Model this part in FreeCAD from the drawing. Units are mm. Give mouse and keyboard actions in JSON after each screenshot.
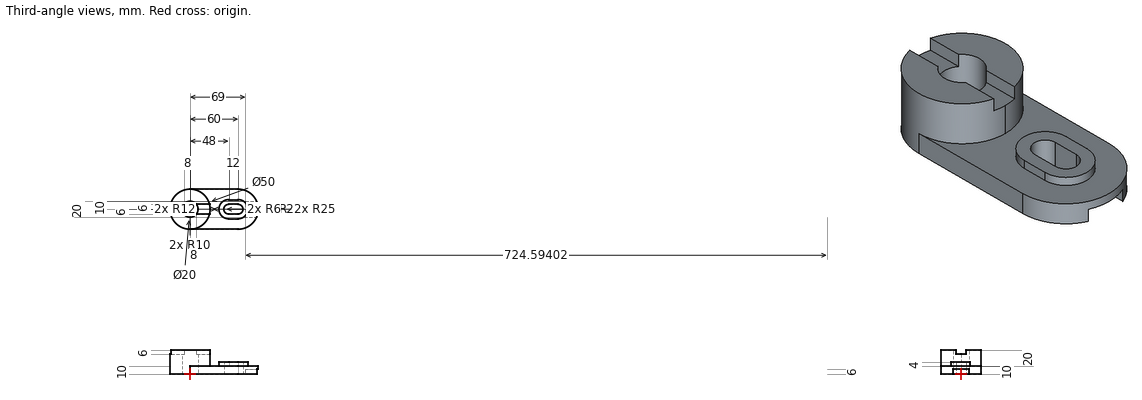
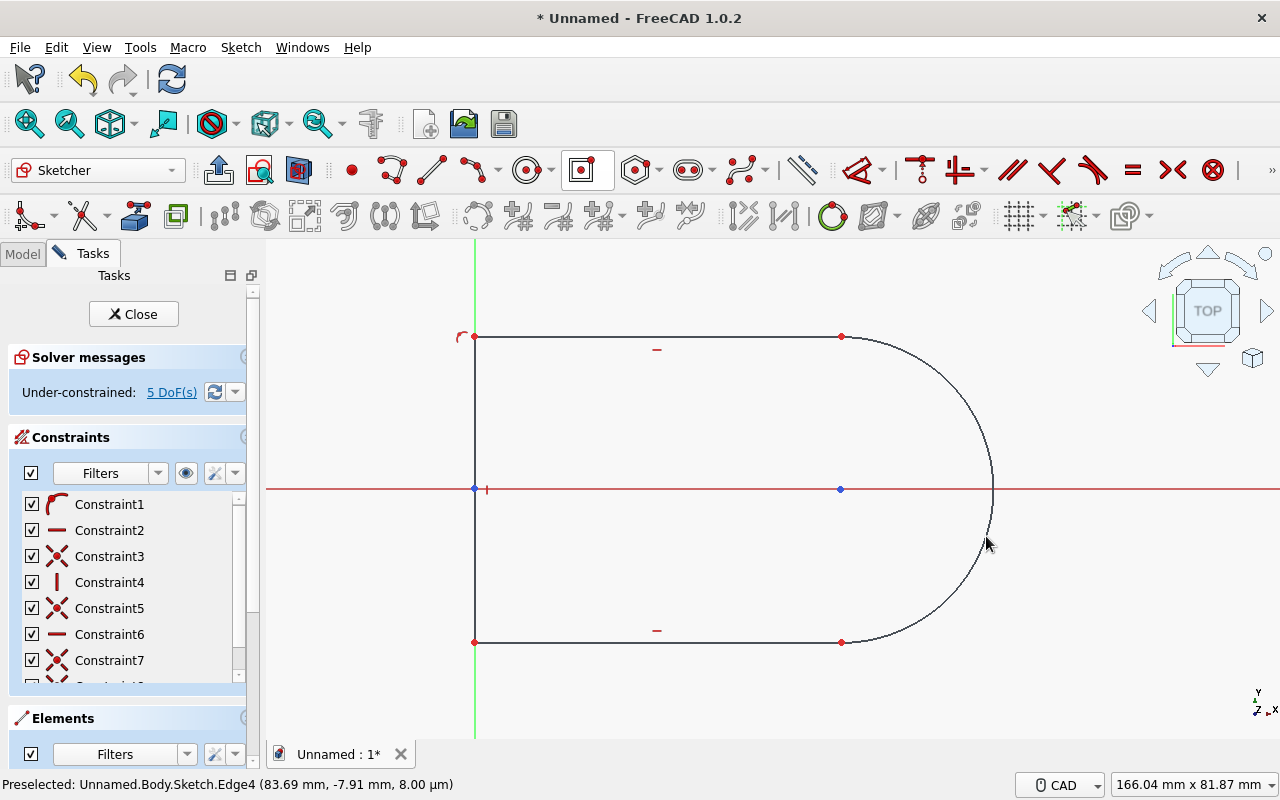
{"action": "left_click", "coordinate": [731, 337]}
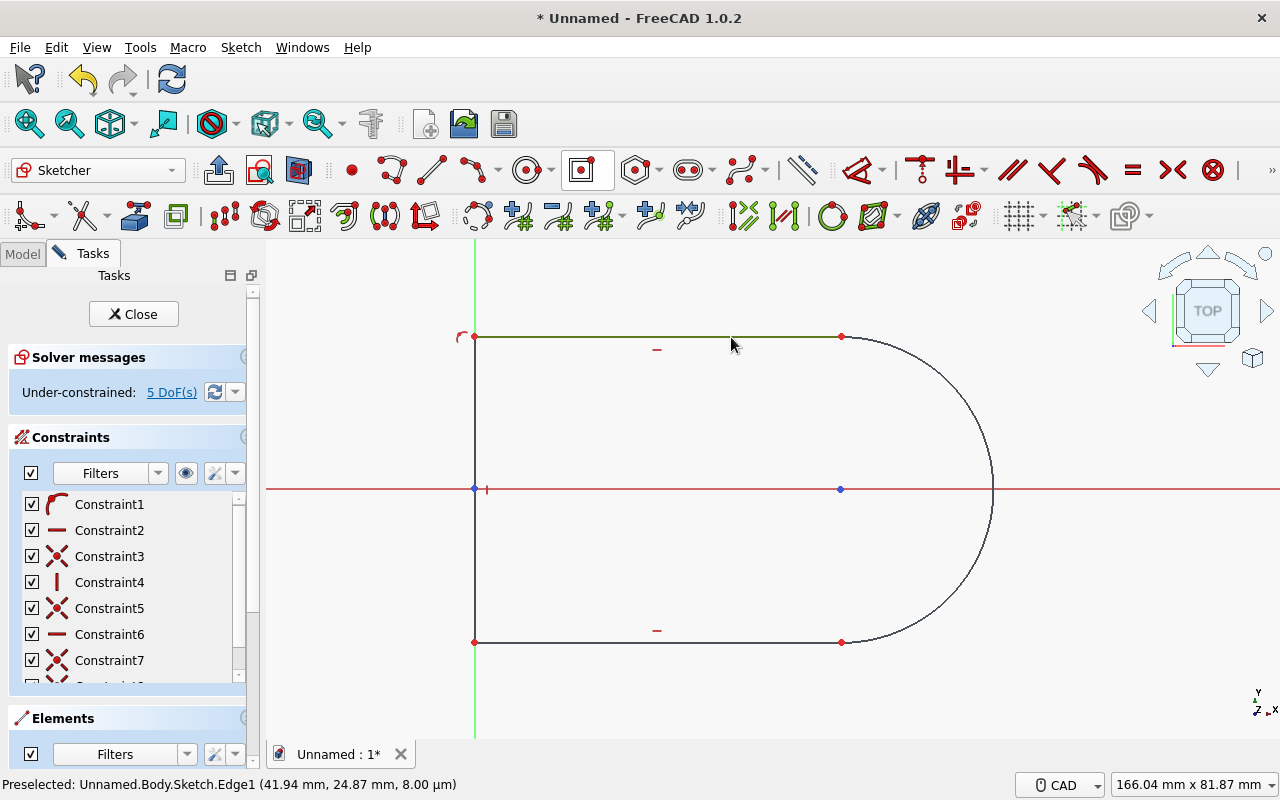
{"action": "left_click", "coordinate": [964, 580]}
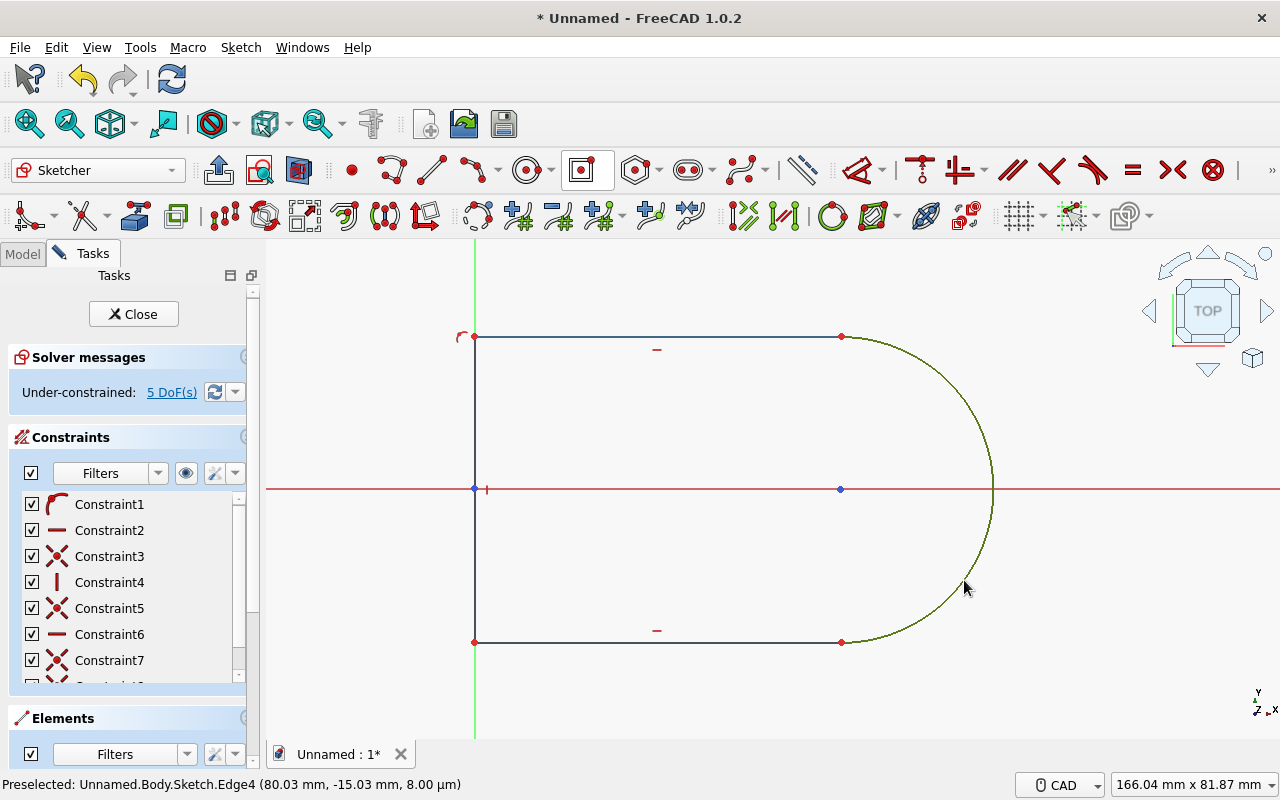
{"action": "left_click", "coordinate": [1094, 170]}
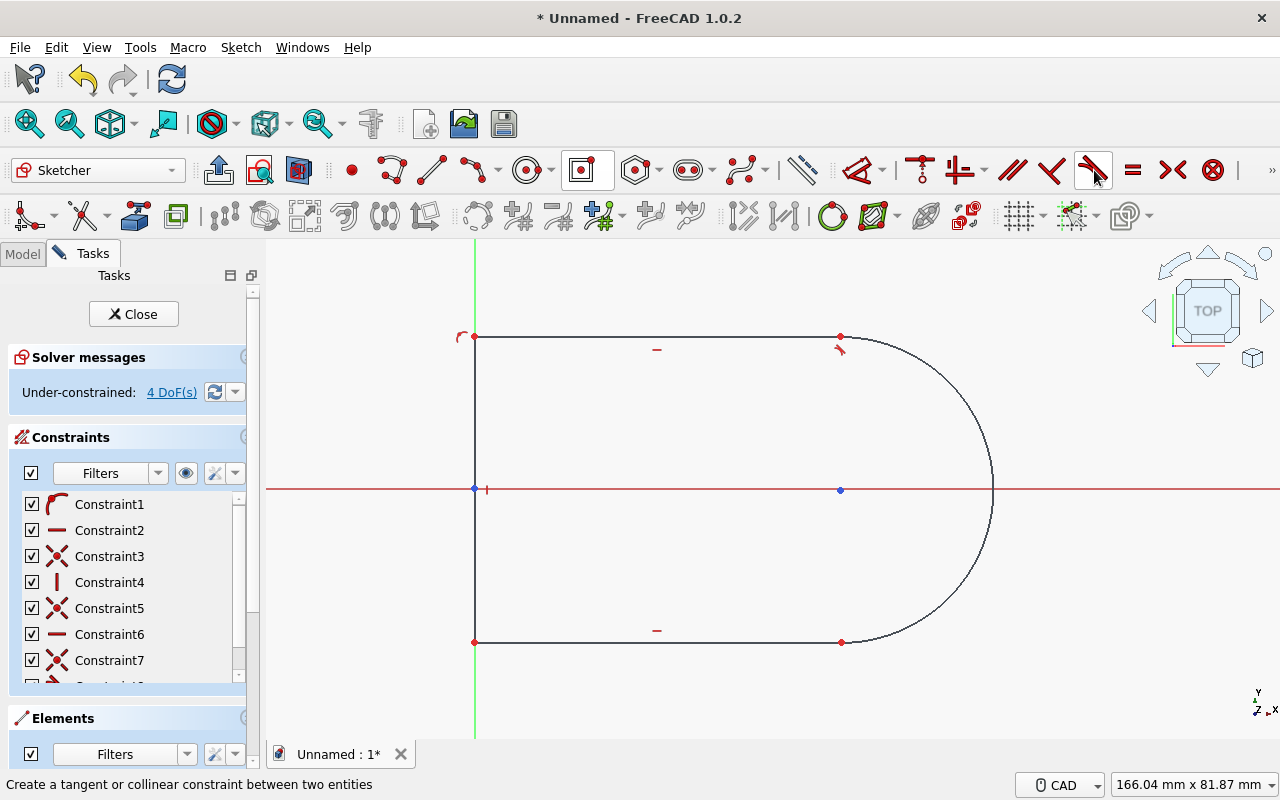
{"action": "left_click", "coordinate": [585, 643]}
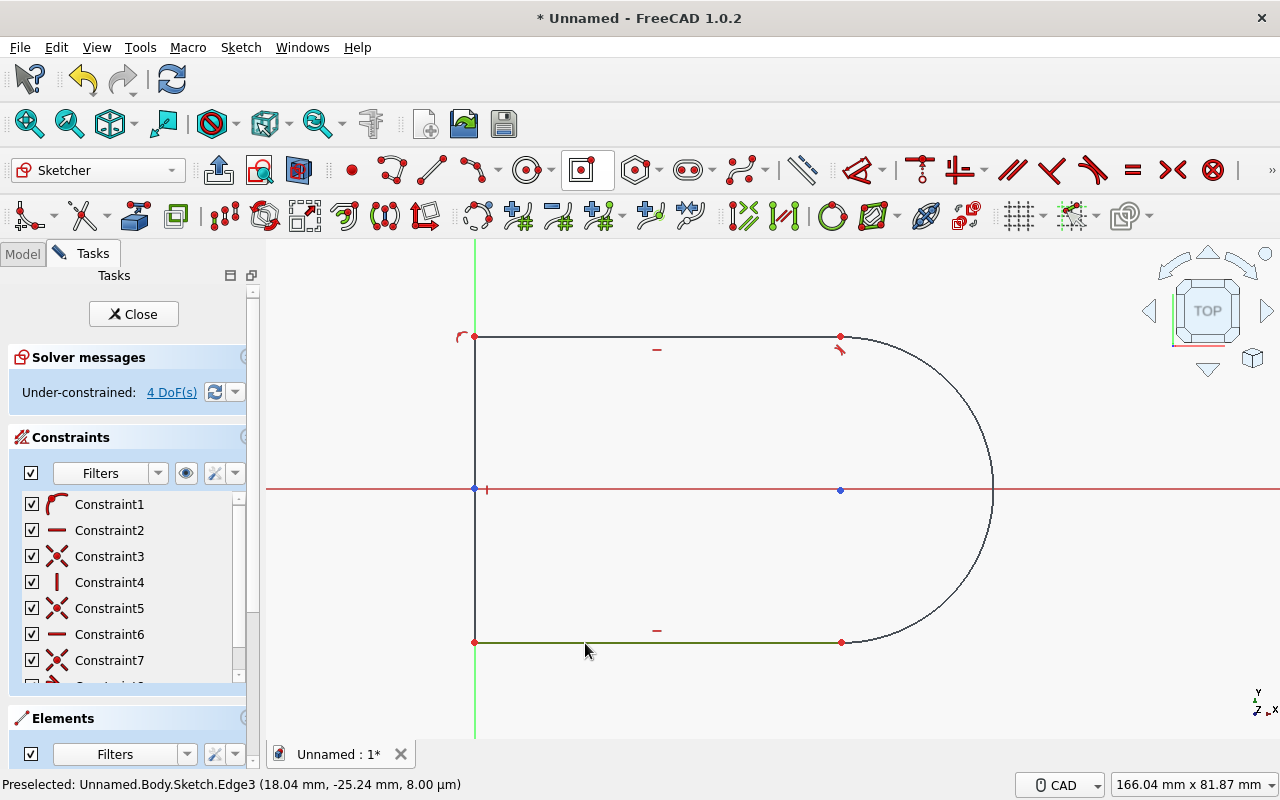
{"action": "left_click", "coordinate": [964, 580]}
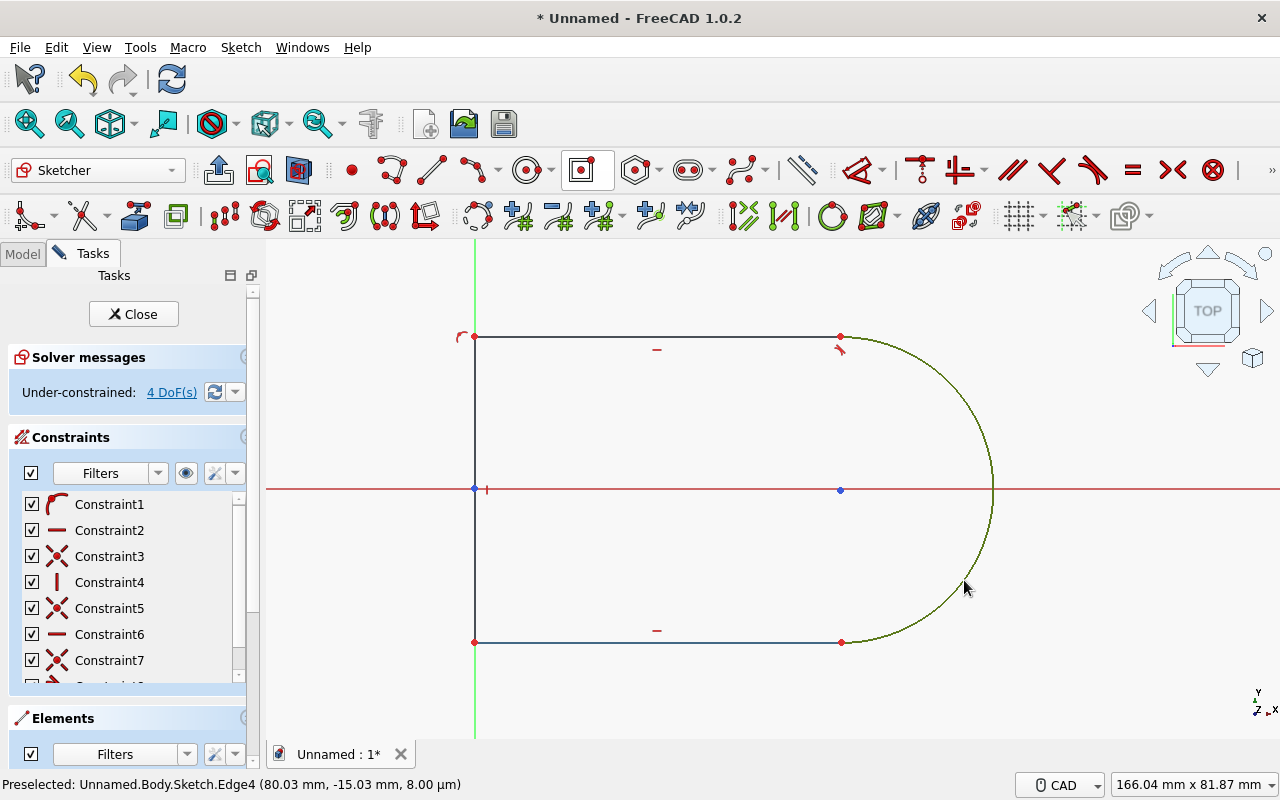
{"action": "left_click", "coordinate": [1094, 170]}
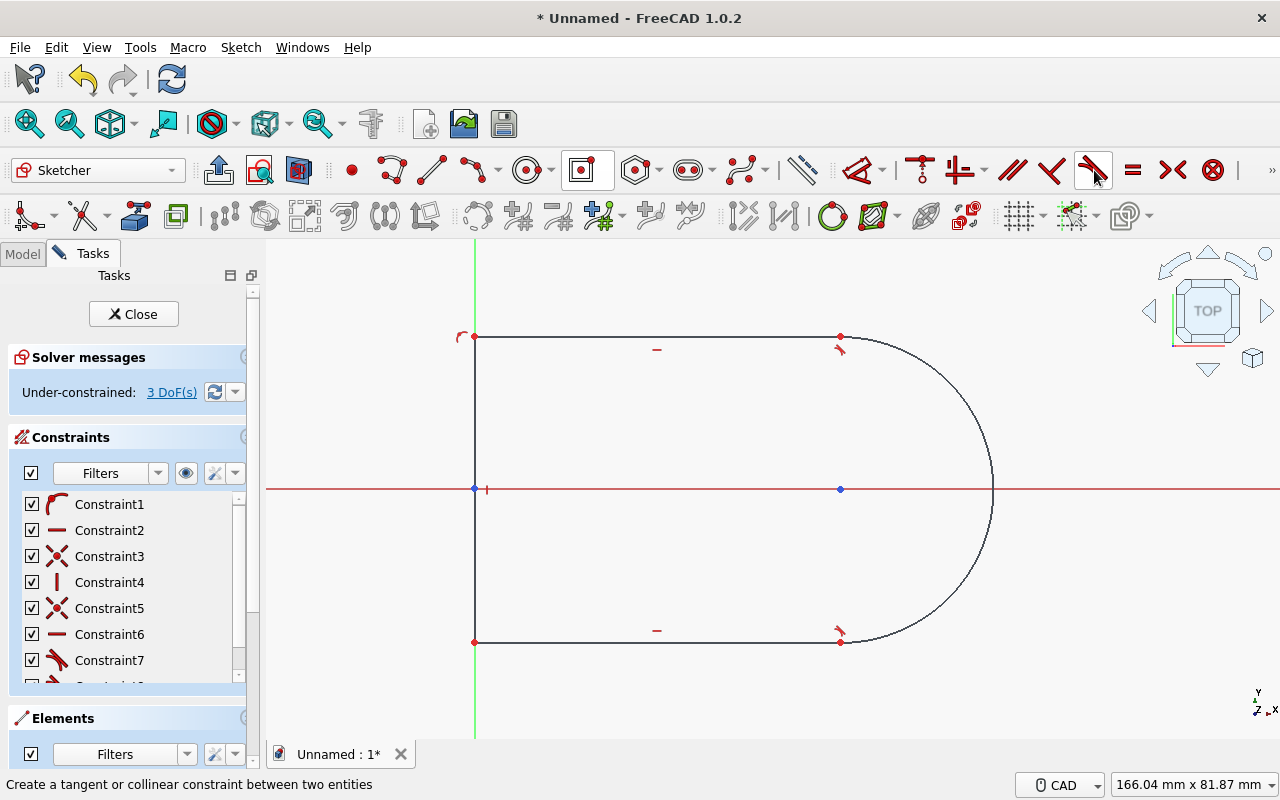
{"action": "left_click", "coordinate": [840, 490]}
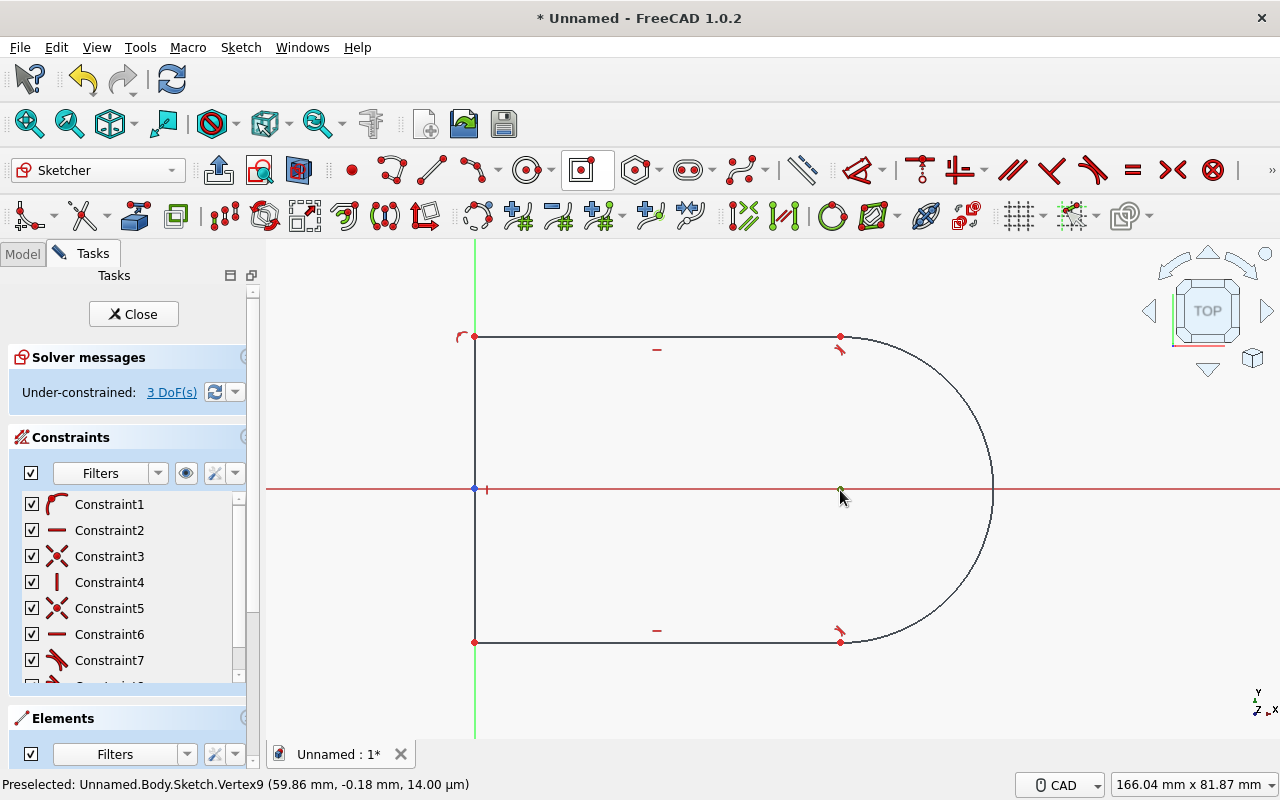
{"action": "left_click", "coordinate": [353, 489]}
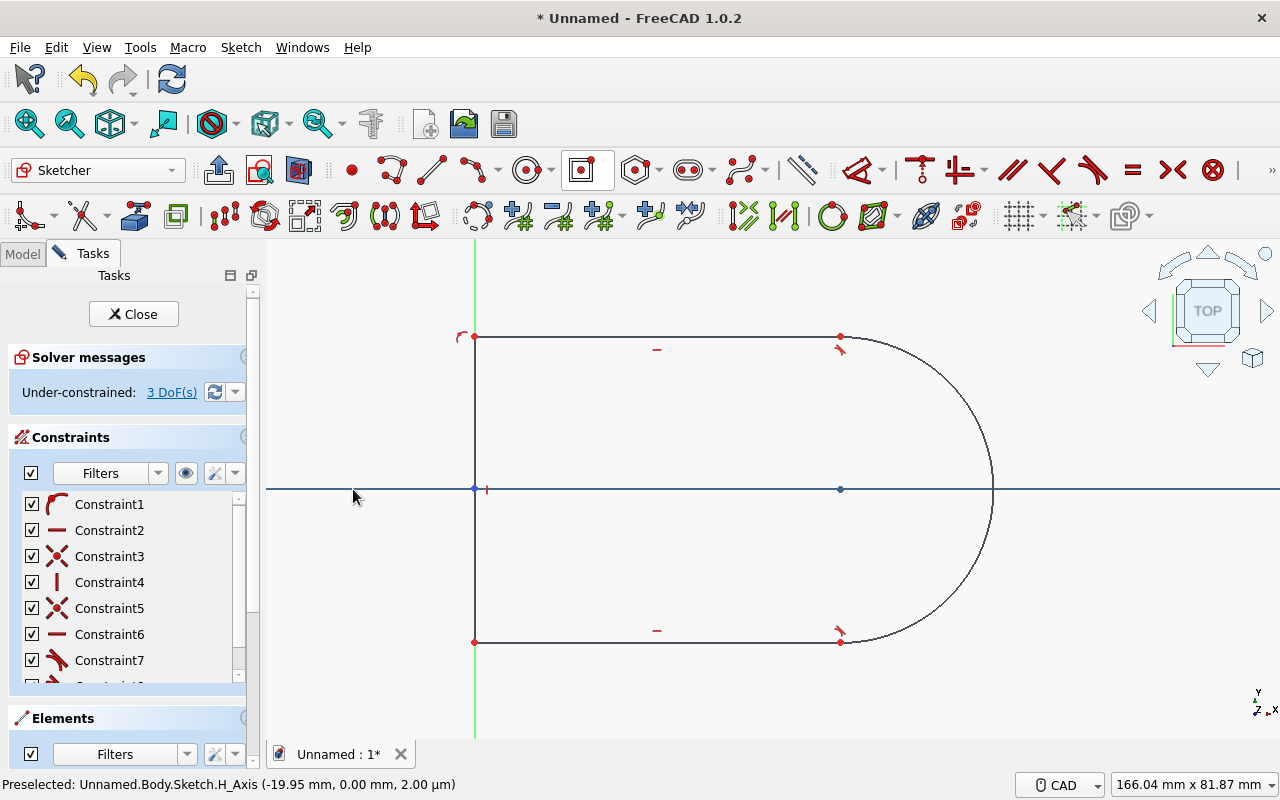
{"action": "left_click", "coordinate": [920, 170]}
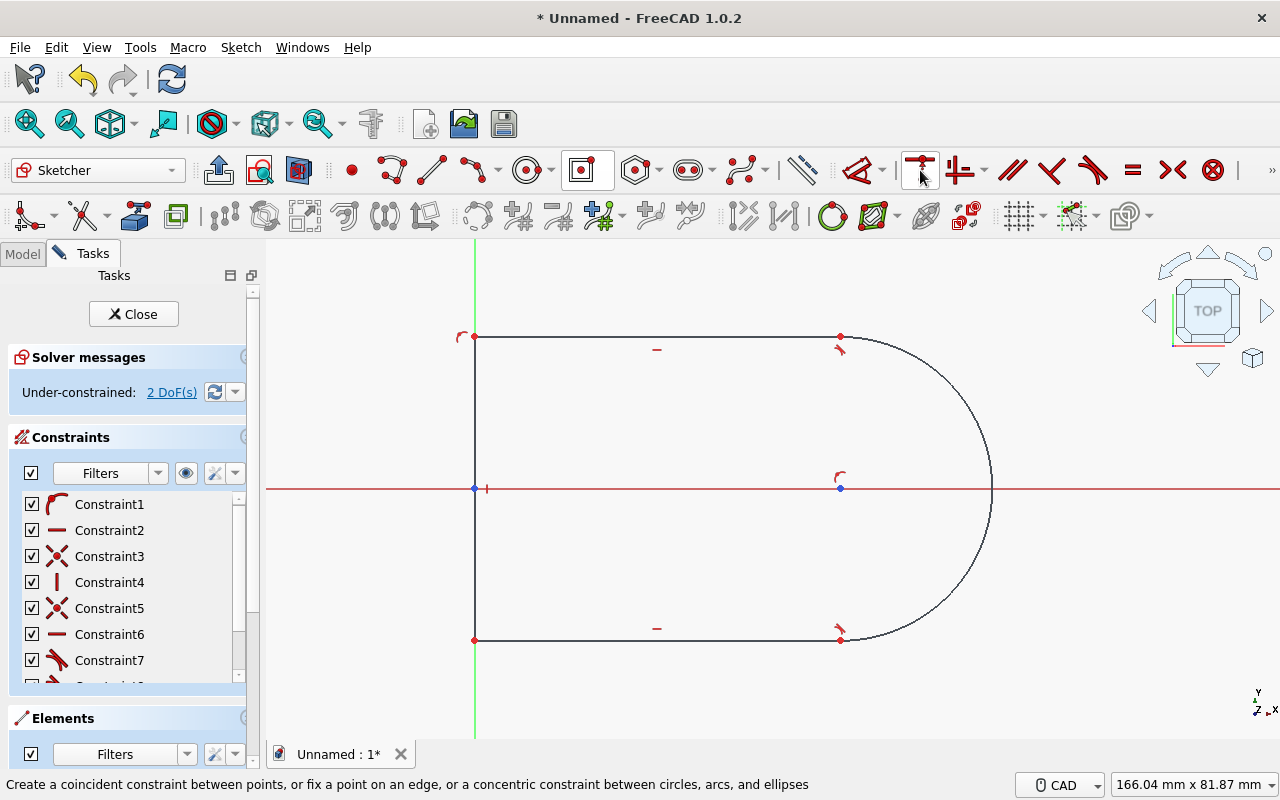
{"action": "left_click", "coordinate": [858, 170]}